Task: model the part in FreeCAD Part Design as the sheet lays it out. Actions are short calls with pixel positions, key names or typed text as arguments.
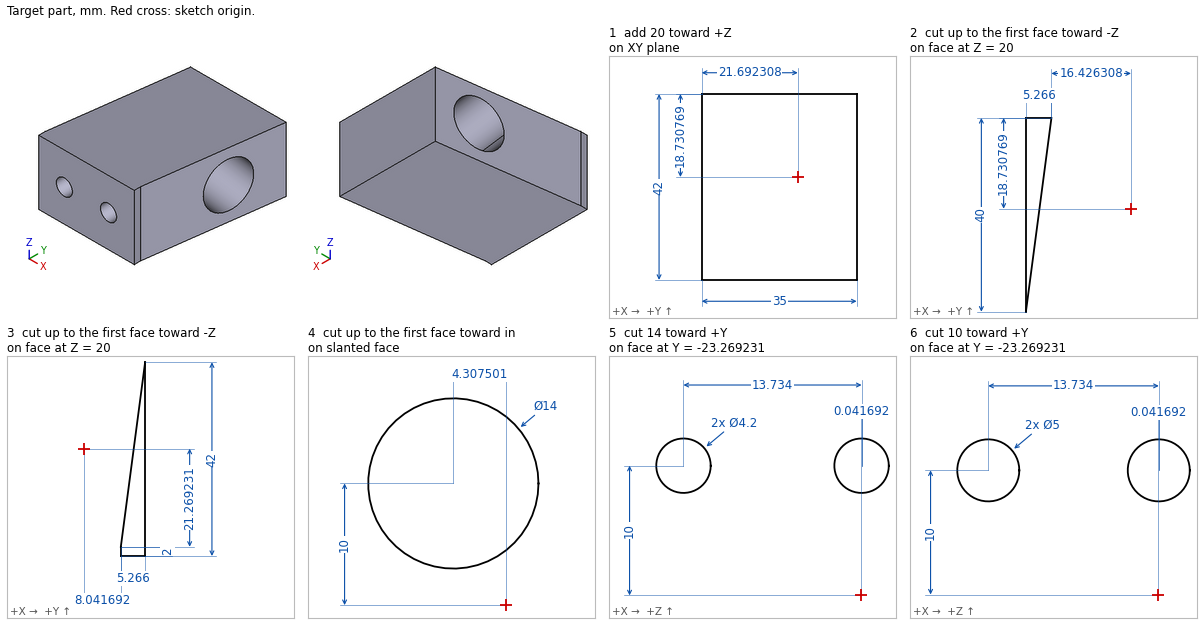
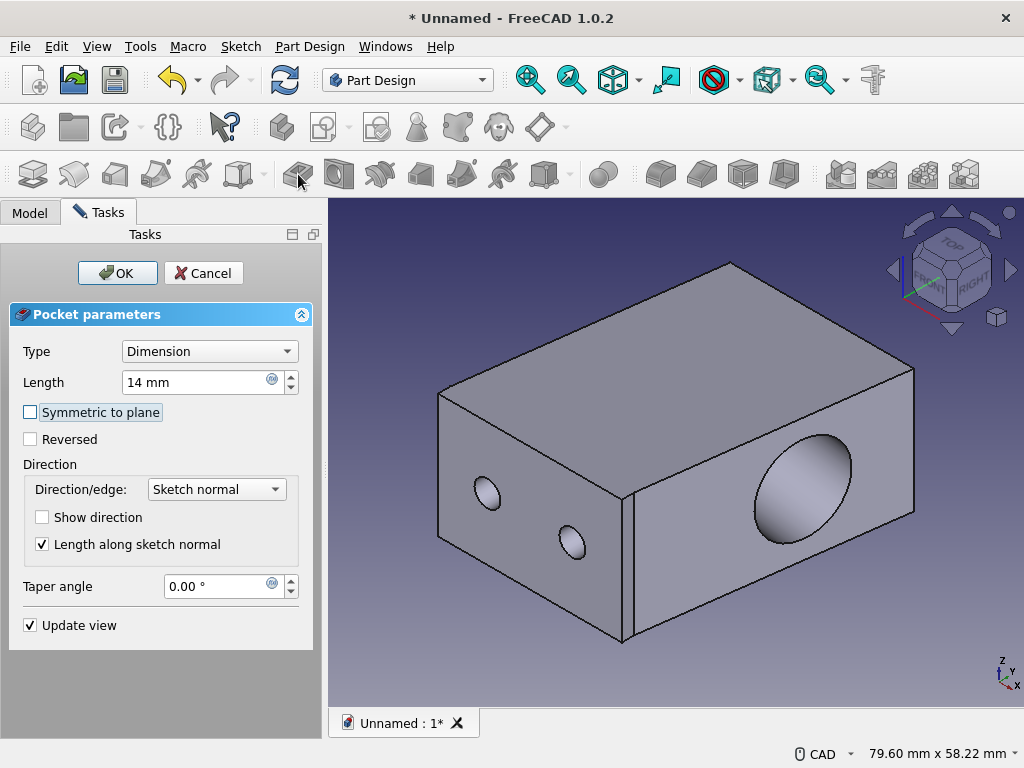
click(118, 273)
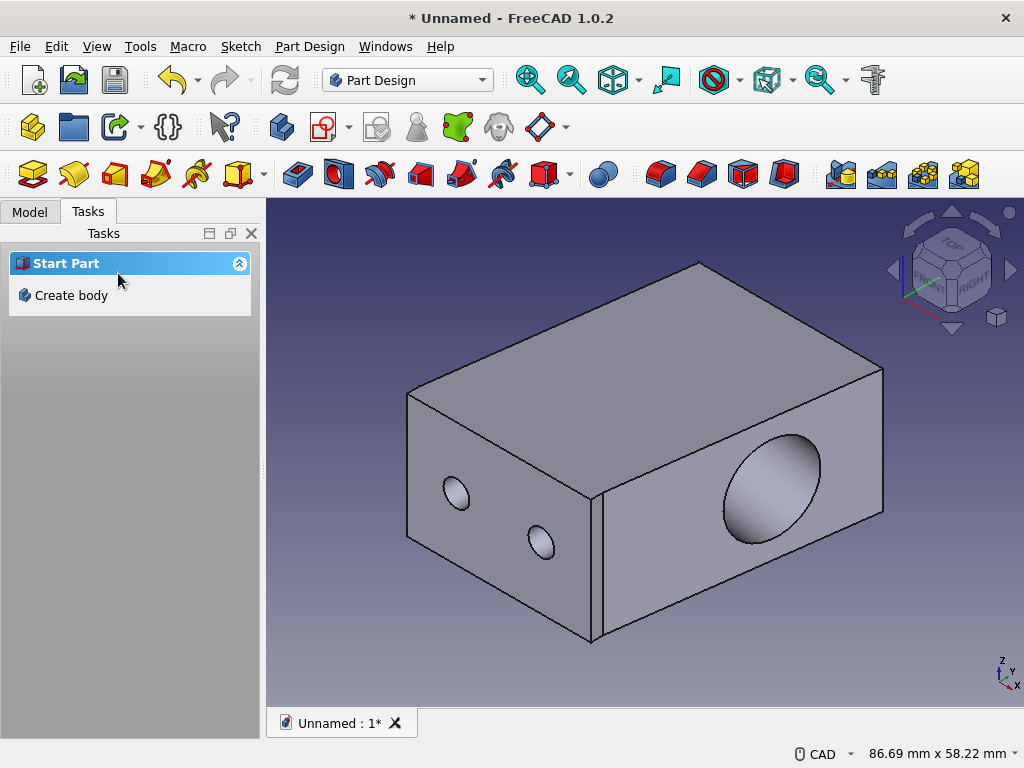
click(499, 497)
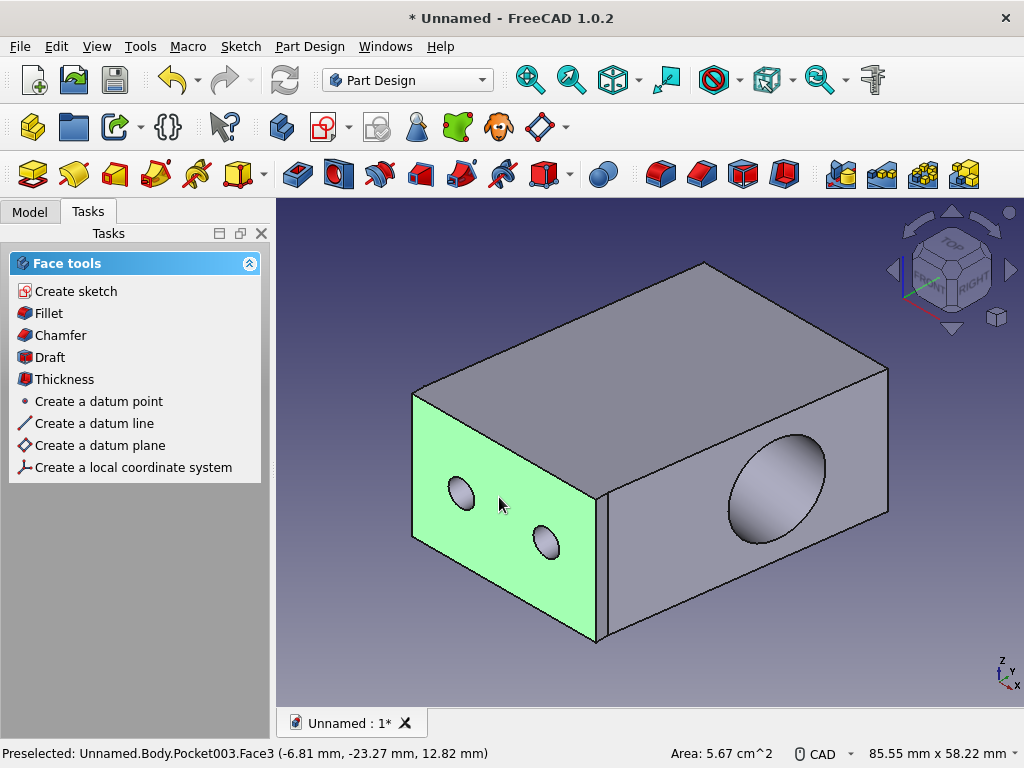
click(322, 128)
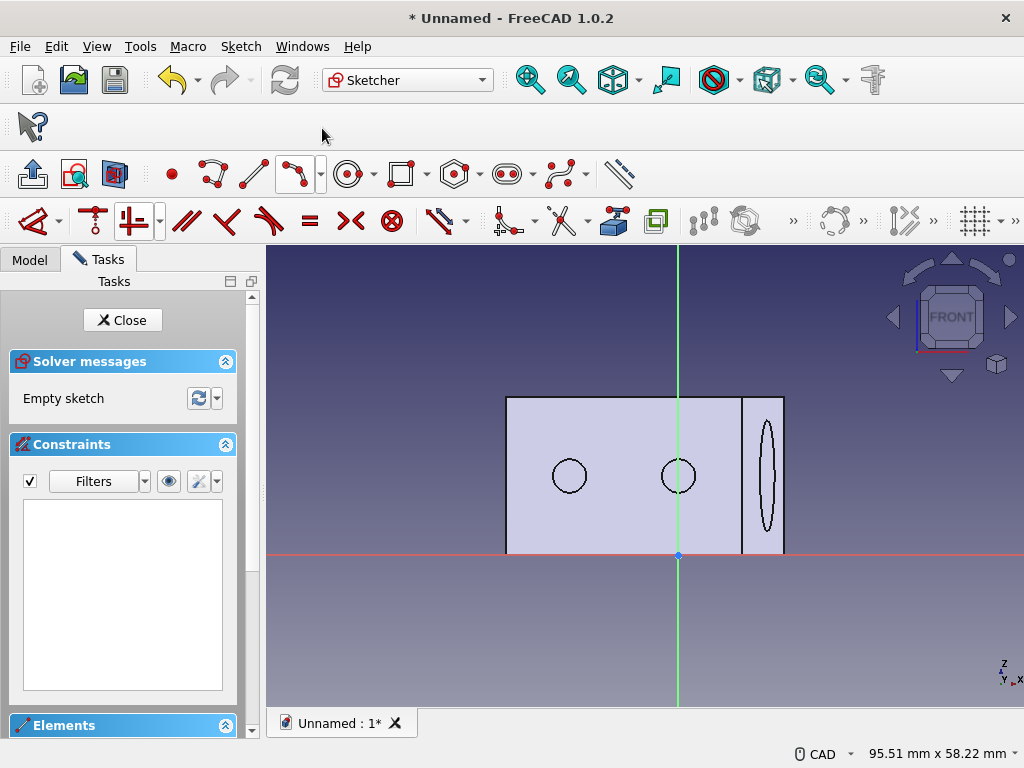
scroll(652, 523, up, 5)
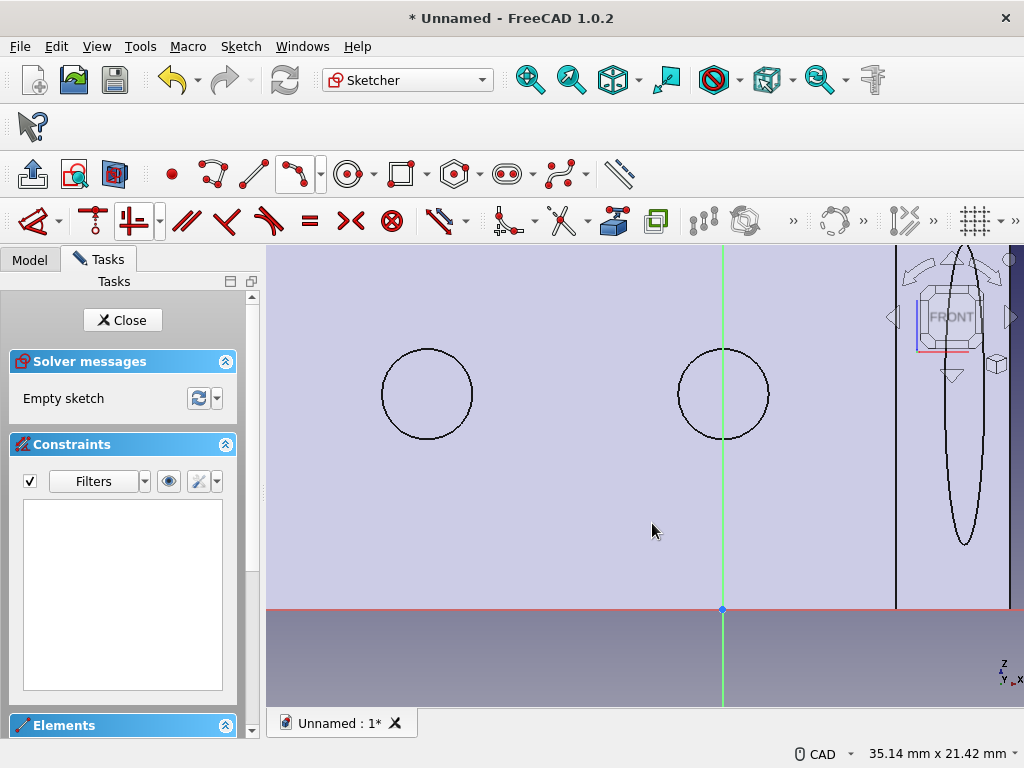
click(348, 174)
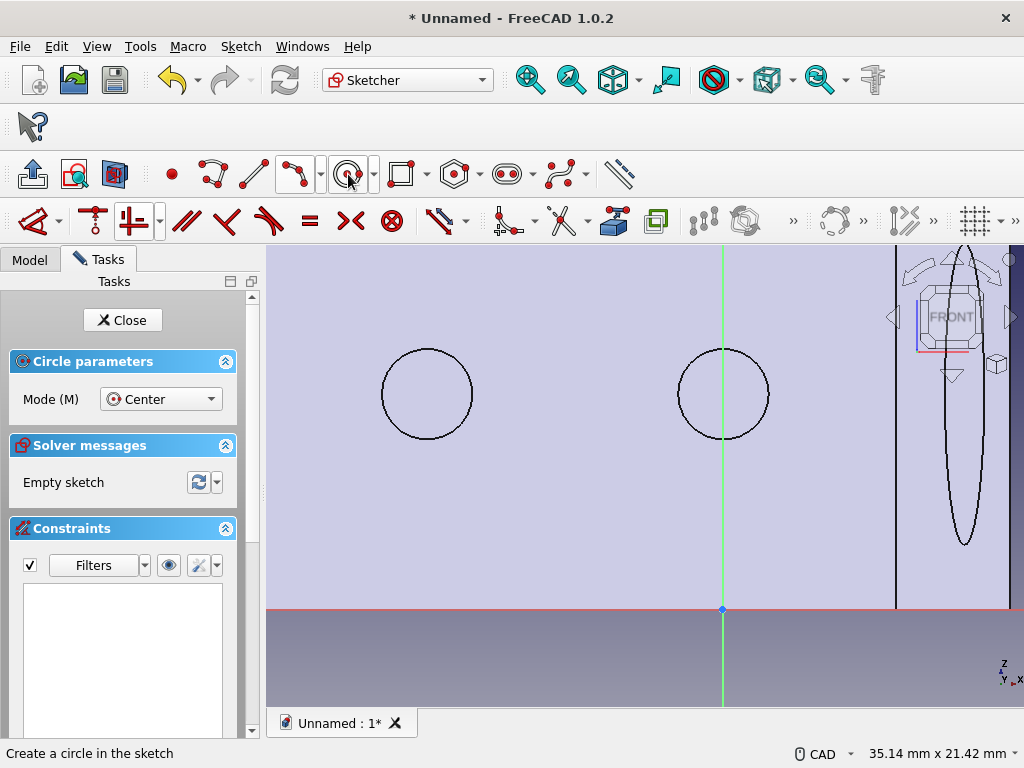
click(427, 394)
click(465, 356)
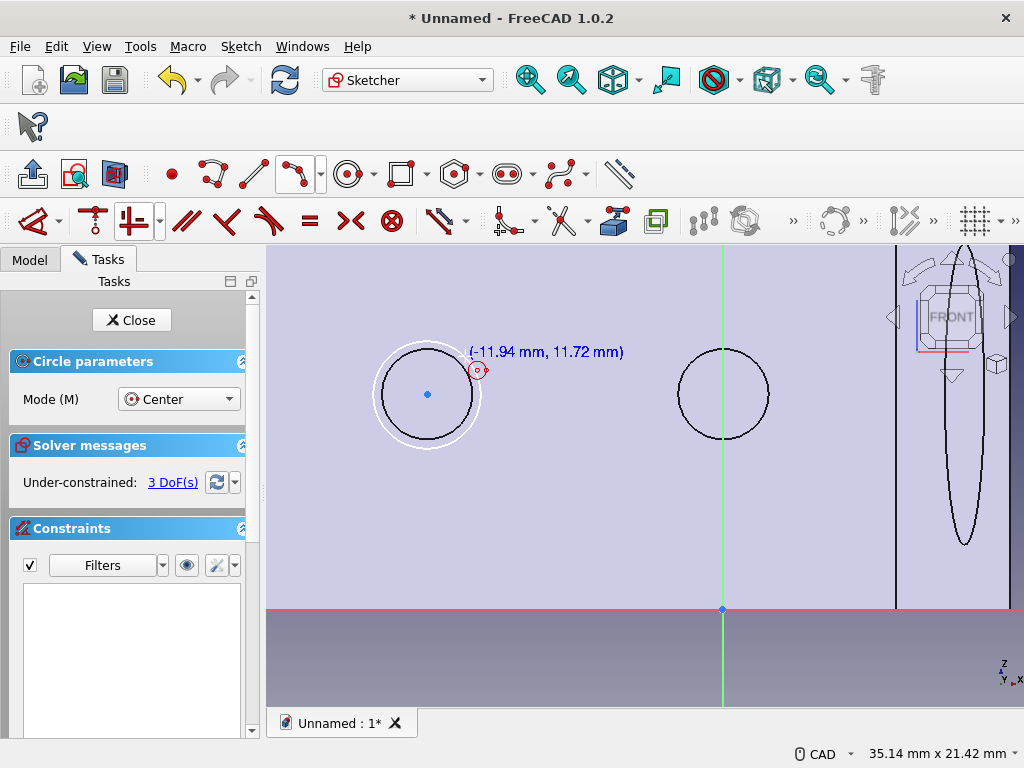
scroll(723, 394, up, 15)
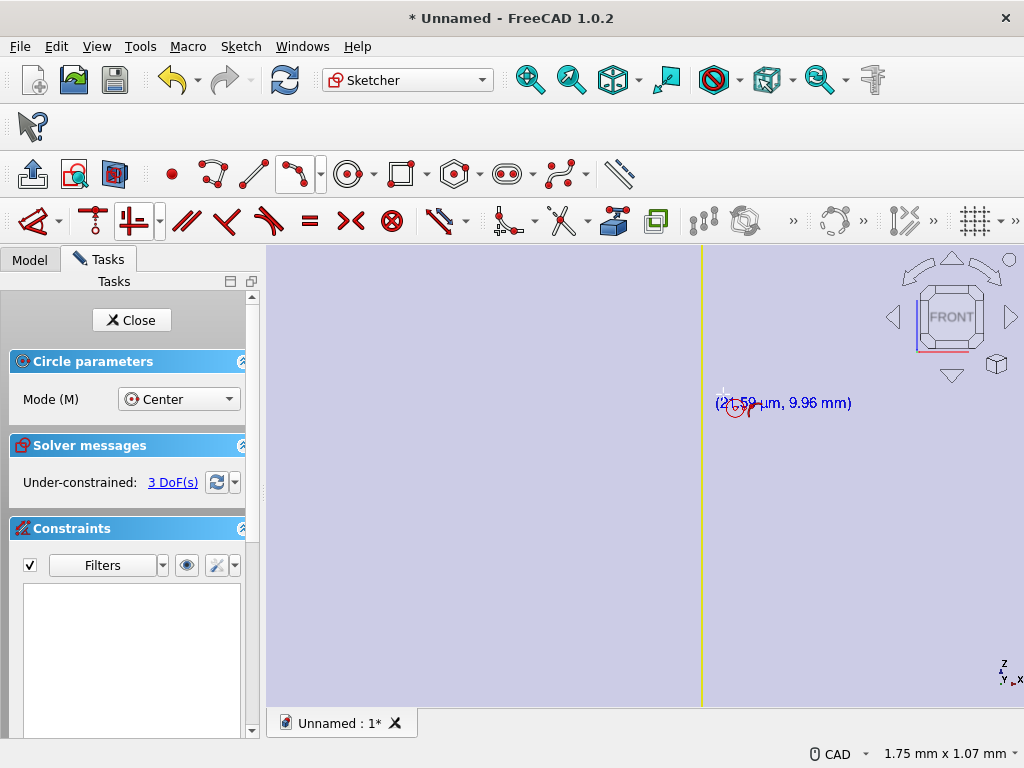
click(720, 392)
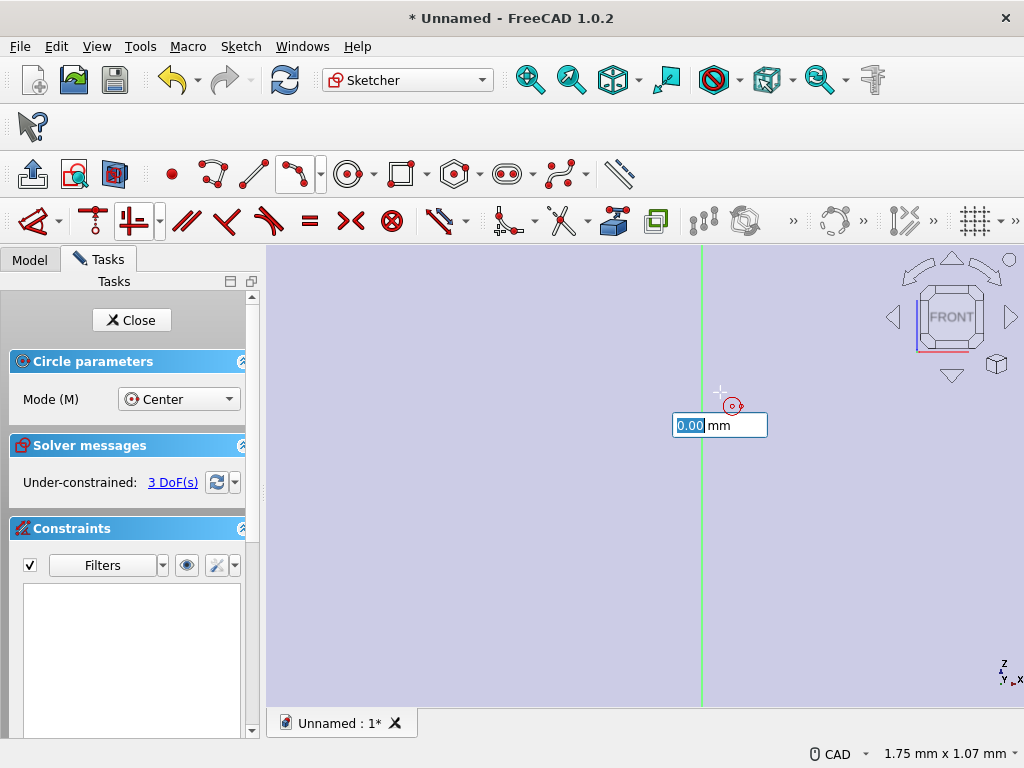
scroll(725, 395, down, 15)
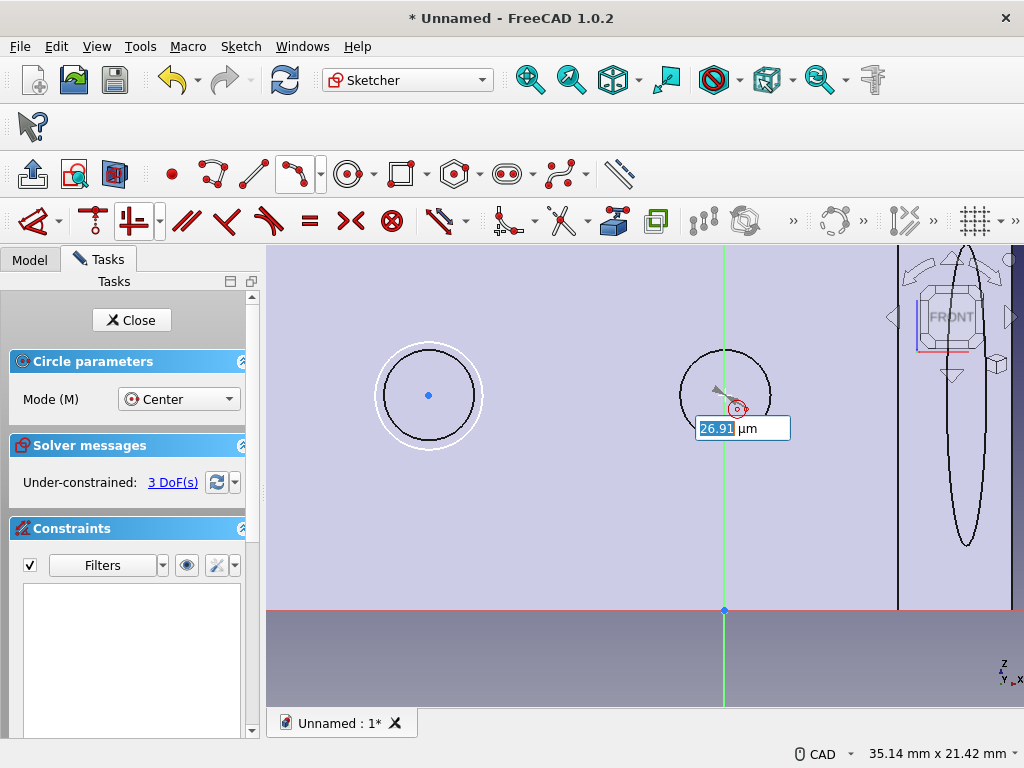
click(763, 357)
key(Escape)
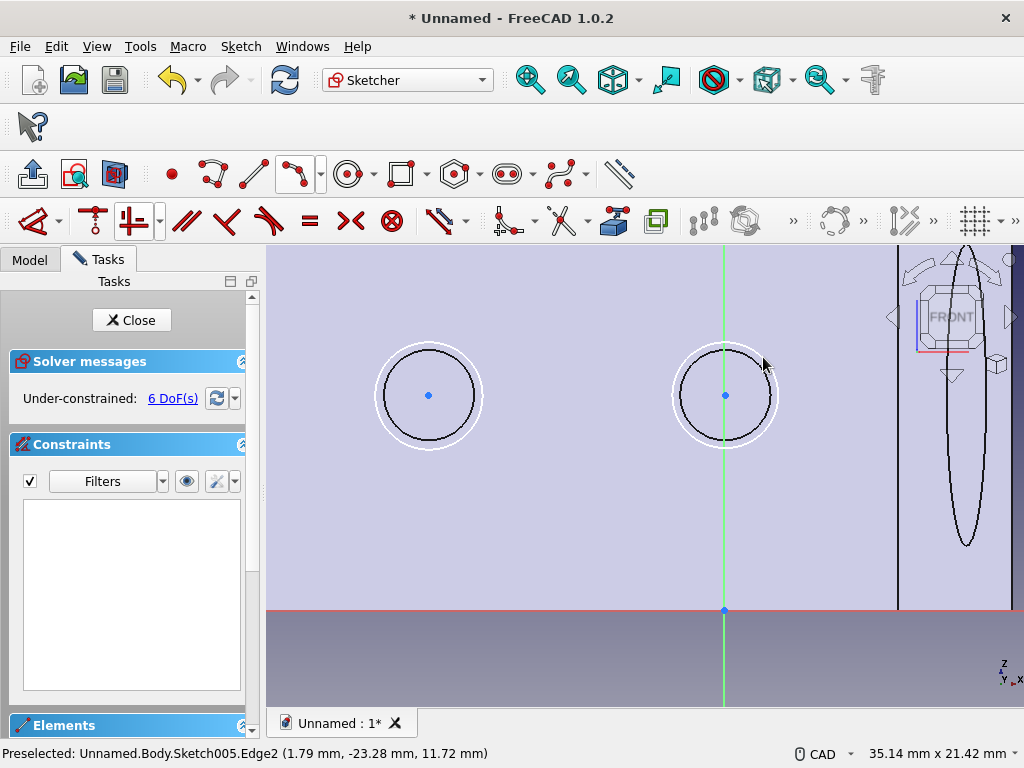
click(467, 358)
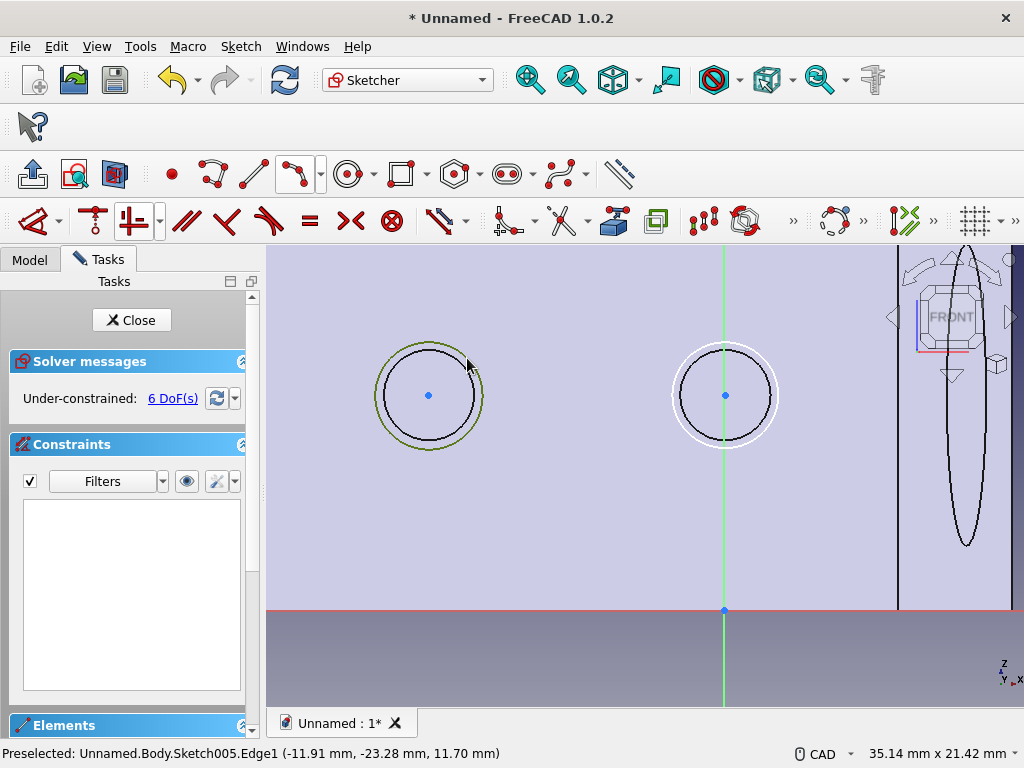
click(763, 358)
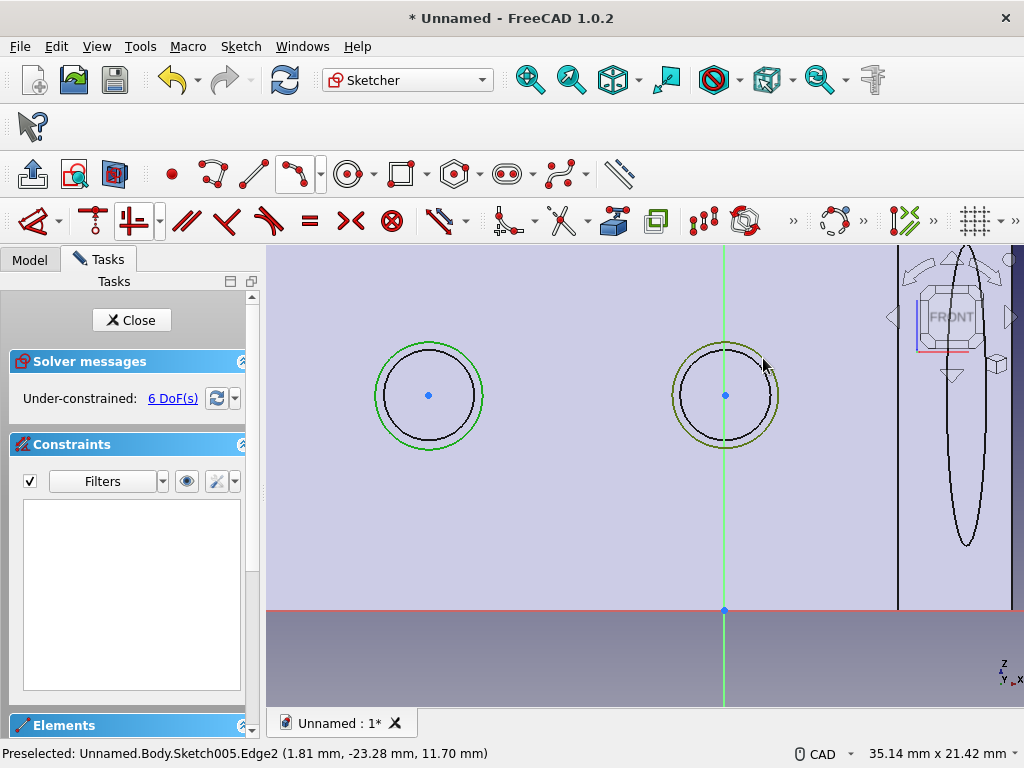
click(310, 222)